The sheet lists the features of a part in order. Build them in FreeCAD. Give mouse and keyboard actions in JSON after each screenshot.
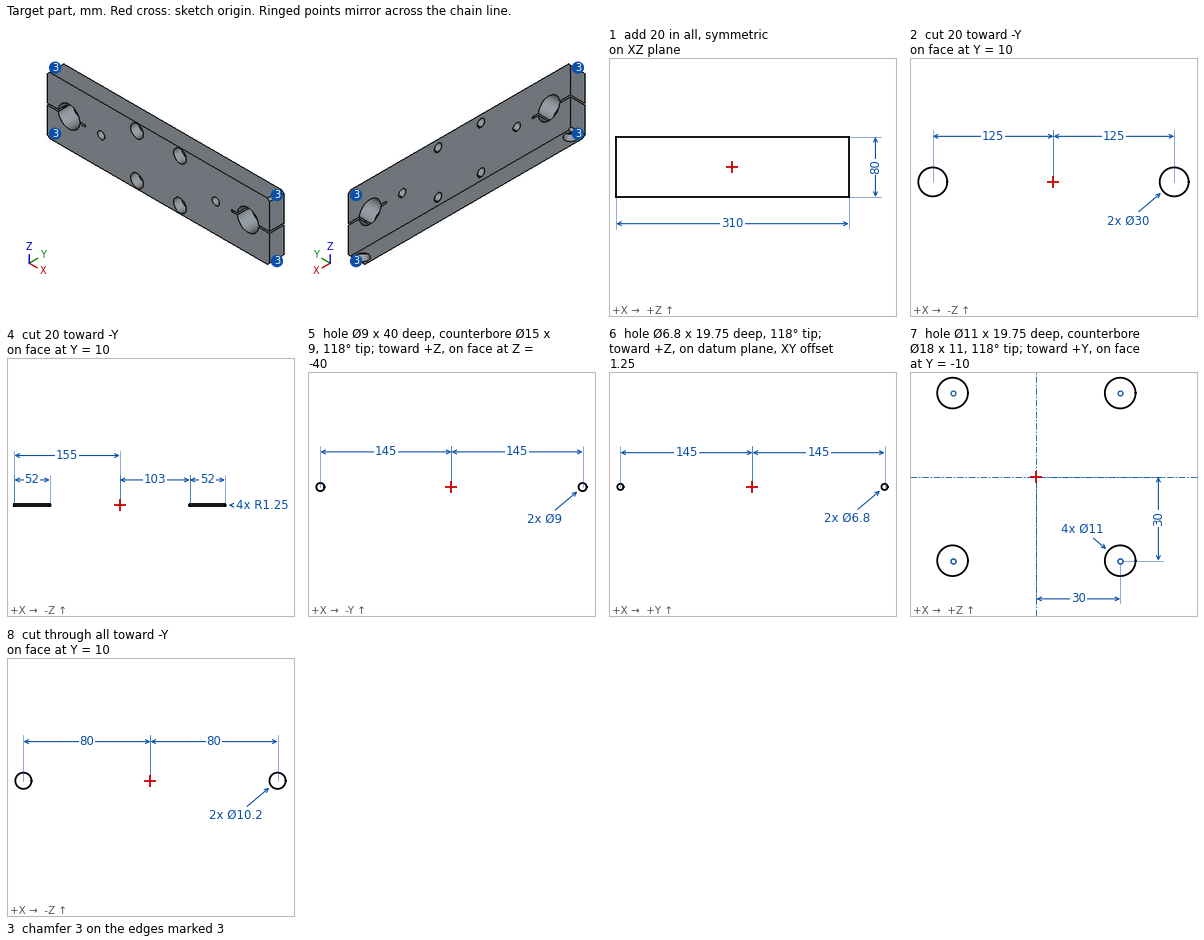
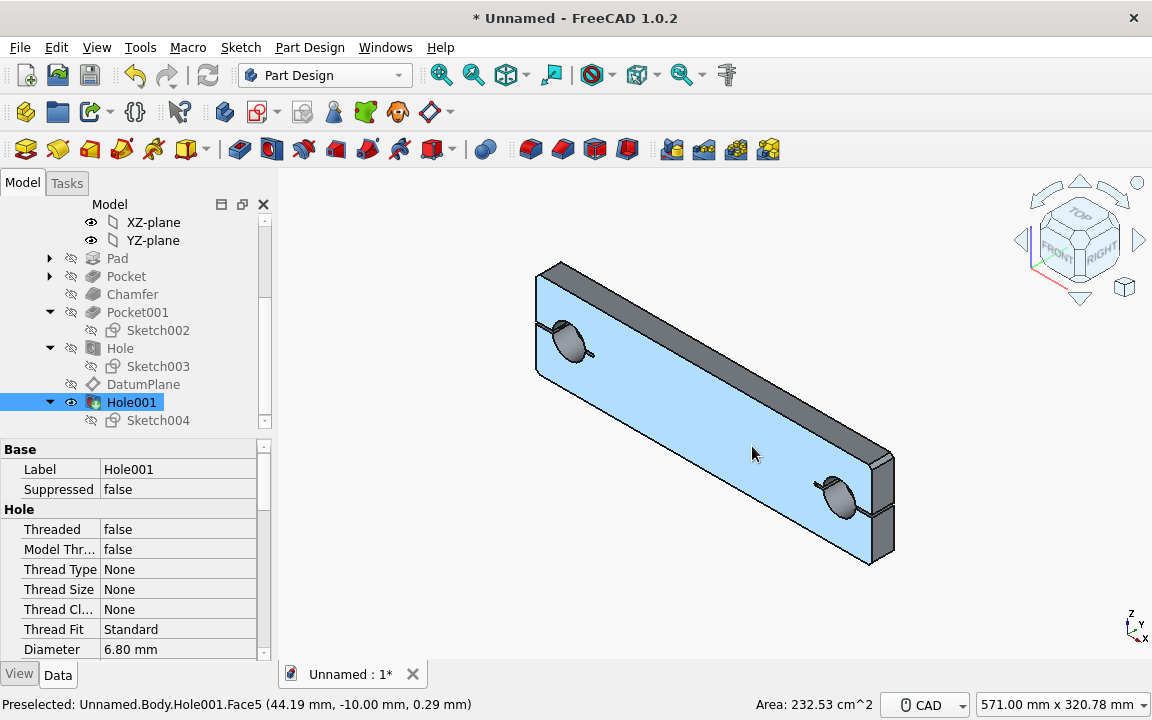
{"action": "left_click", "coordinate": [258, 112]}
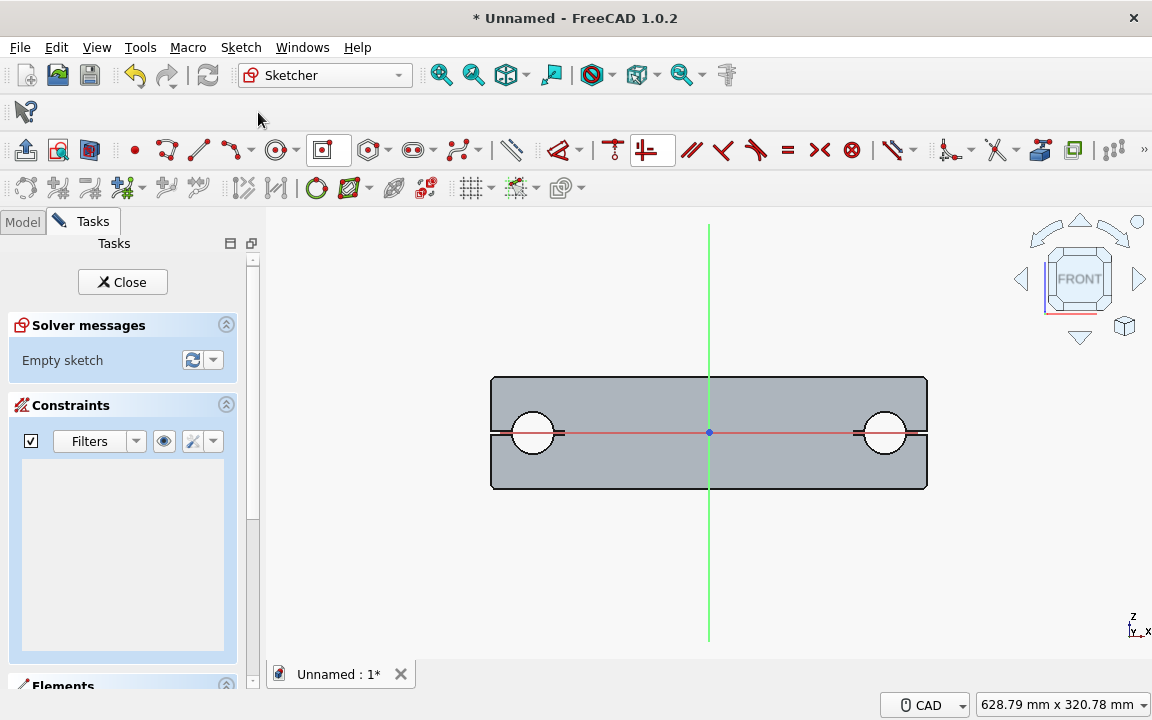
{"action": "scroll", "coordinate": [749, 433], "scroll_direction": "up", "scroll_amount": 5}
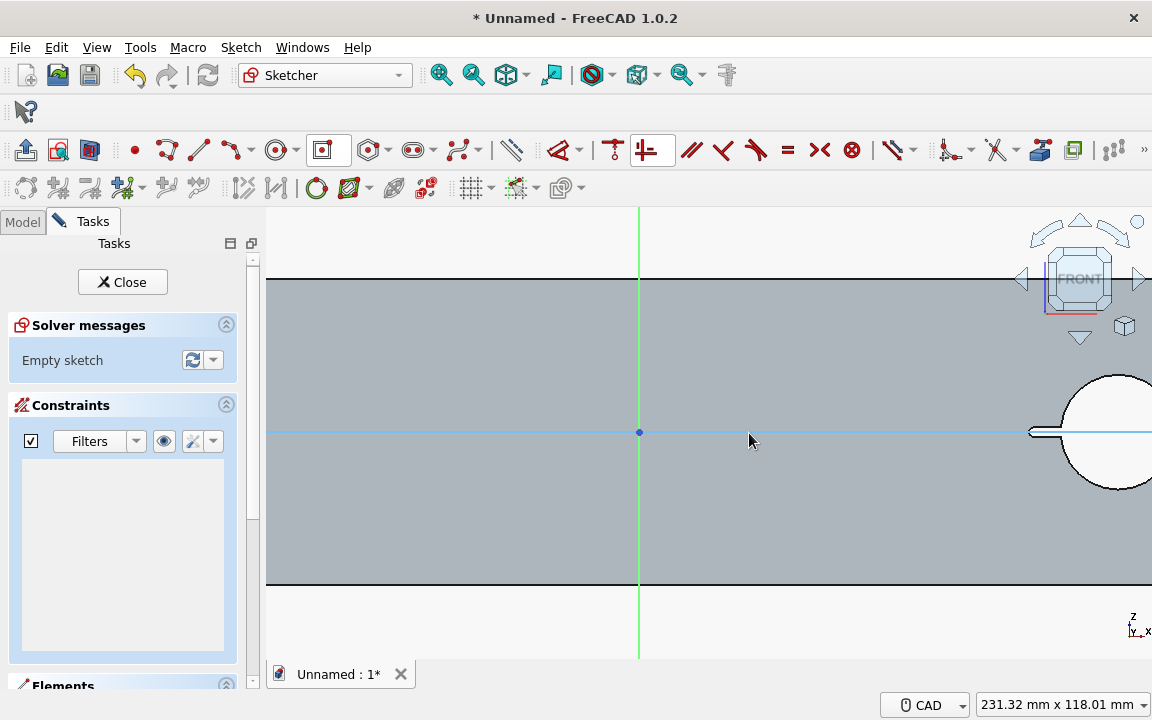
{"action": "left_click", "coordinate": [276, 150]}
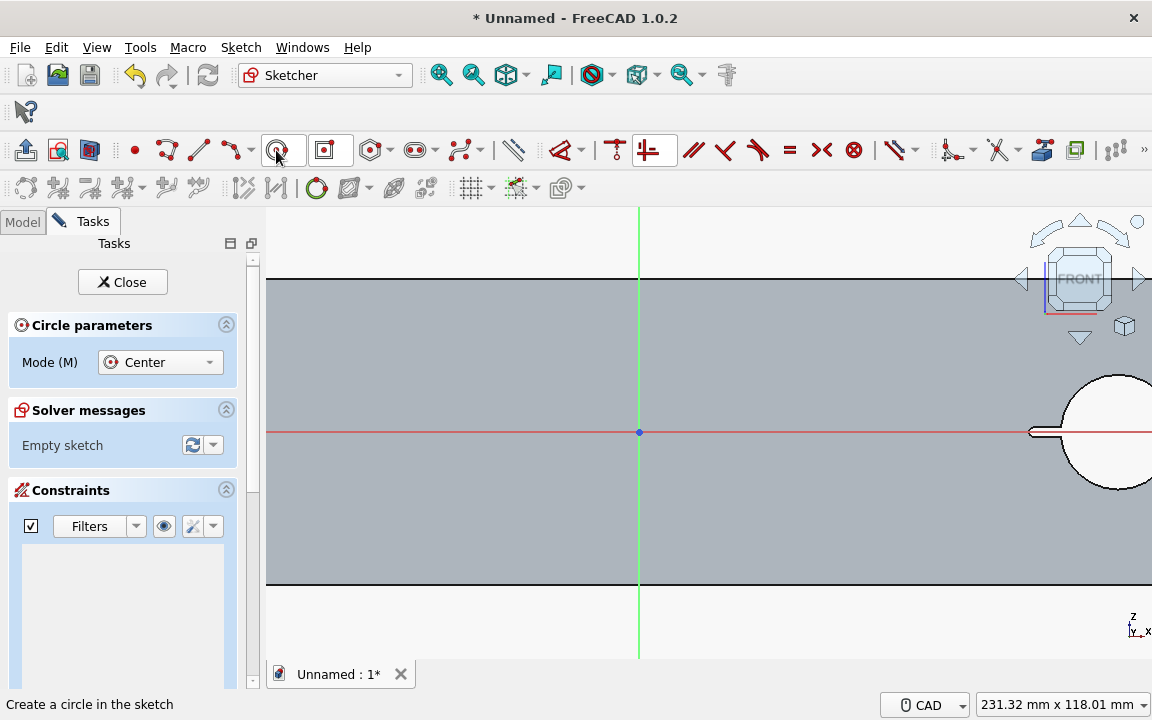
{"action": "left_click", "coordinate": [754, 547]}
{"action": "mouse_move", "coordinate": [769, 532]}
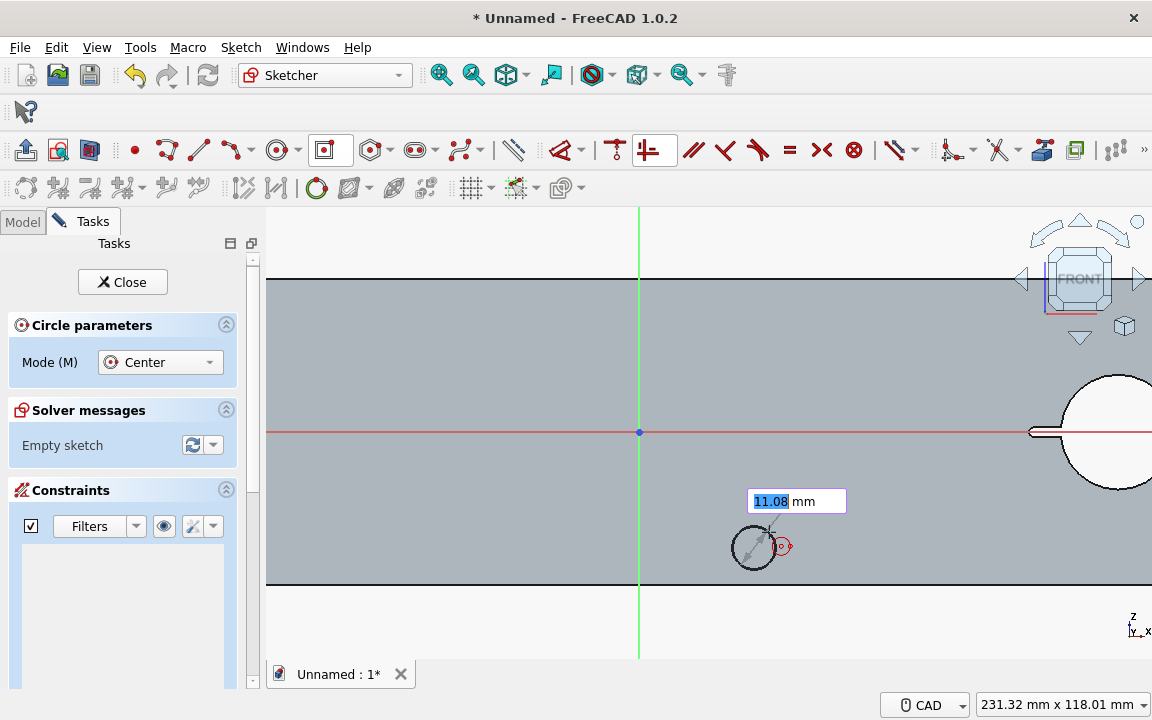
{"action": "type", "text": "11"}
{"action": "key", "text": "Return"}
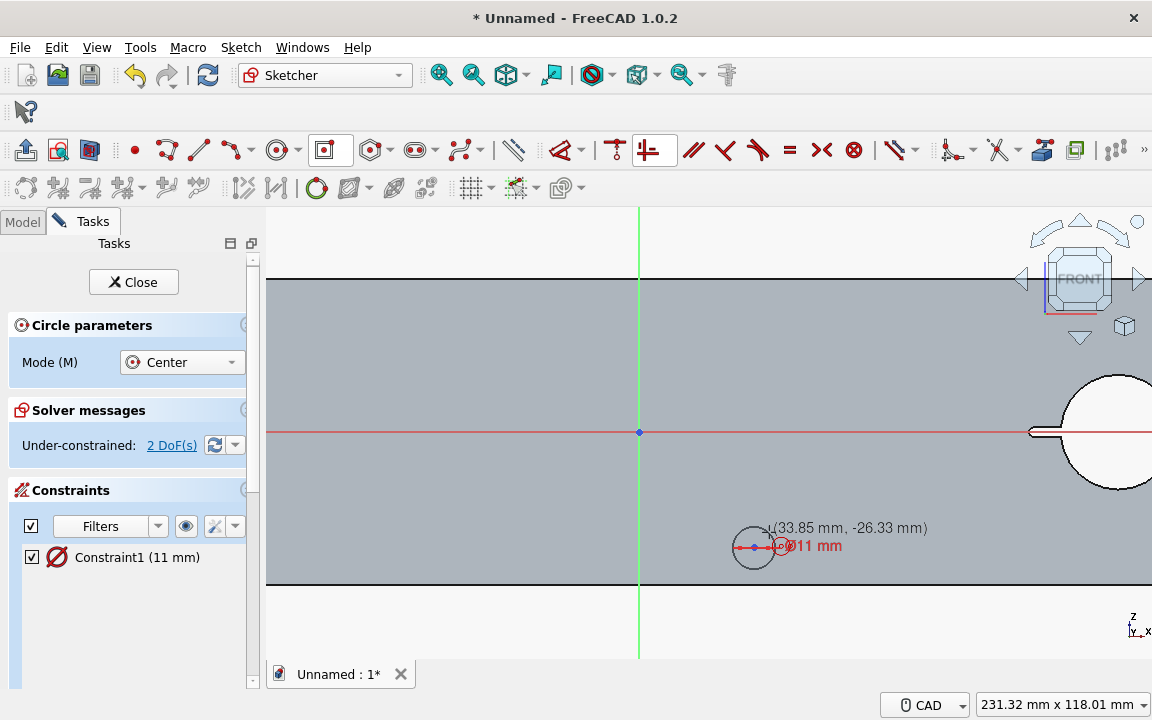
{"action": "left_click", "coordinate": [524, 547]}
{"action": "mouse_move", "coordinate": [539, 532]}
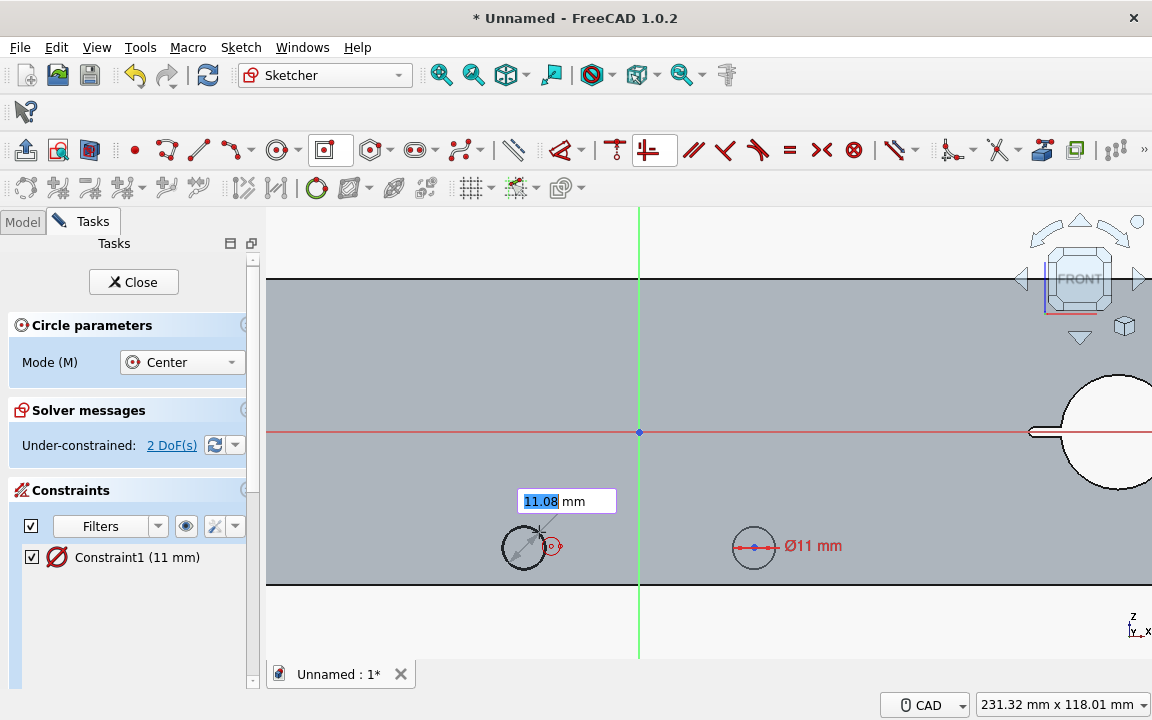
{"action": "type", "text": "11"}
{"action": "key", "text": "Return"}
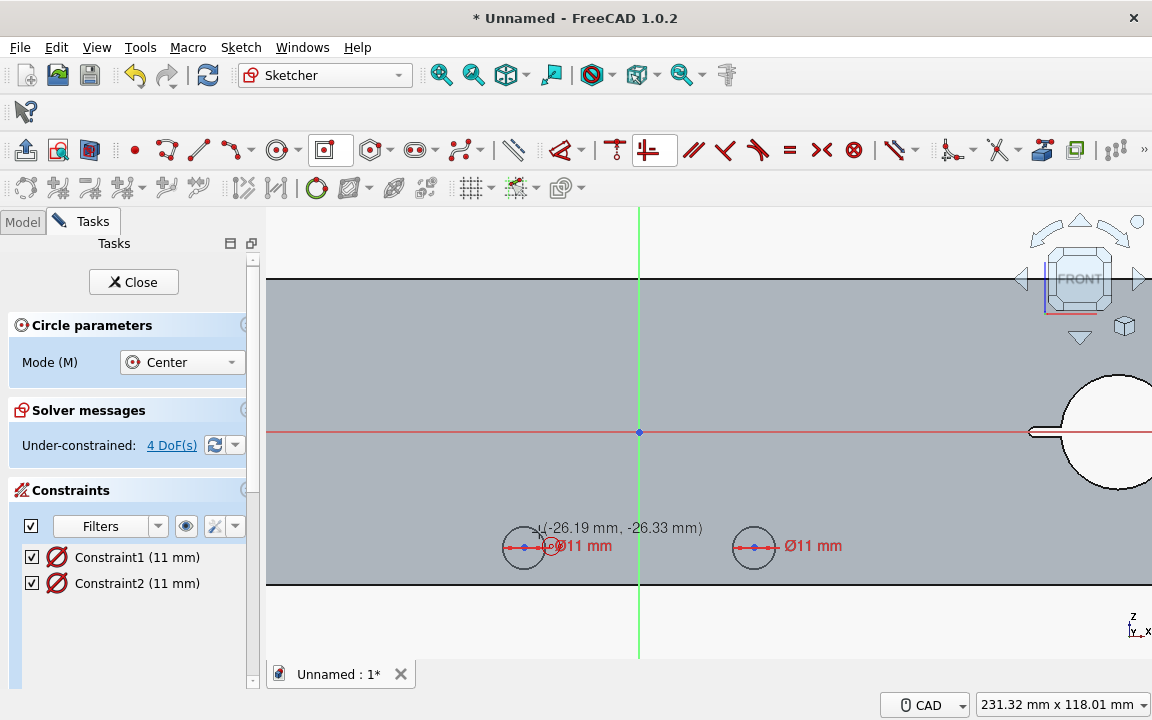
{"action": "left_click", "coordinate": [524, 317]}
{"action": "mouse_move", "coordinate": [539, 302]}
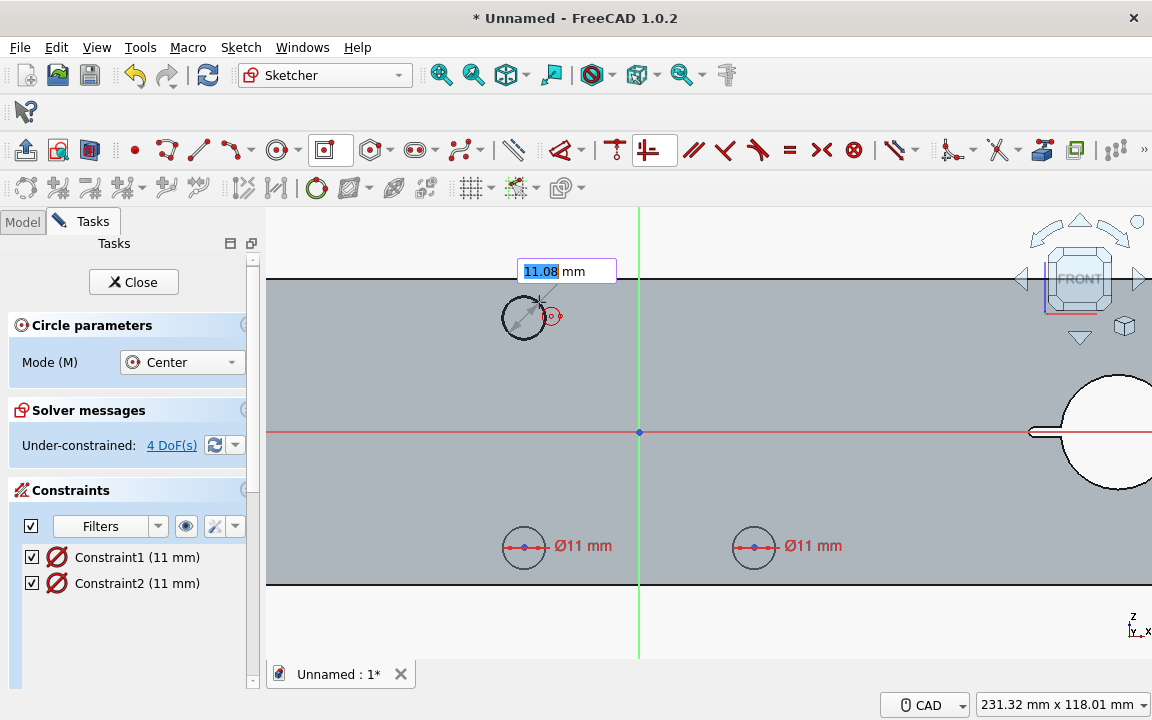
{"action": "type", "text": "11"}
{"action": "key", "text": "Return"}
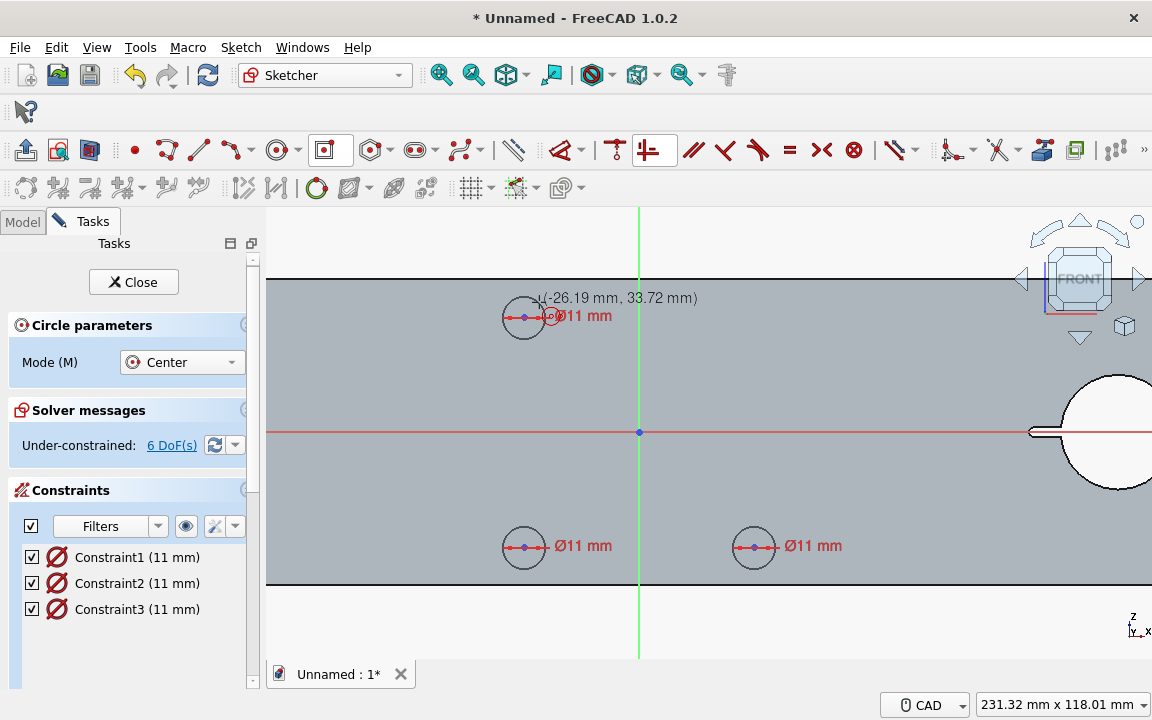
{"action": "left_click", "coordinate": [754, 317]}
{"action": "mouse_move", "coordinate": [769, 302]}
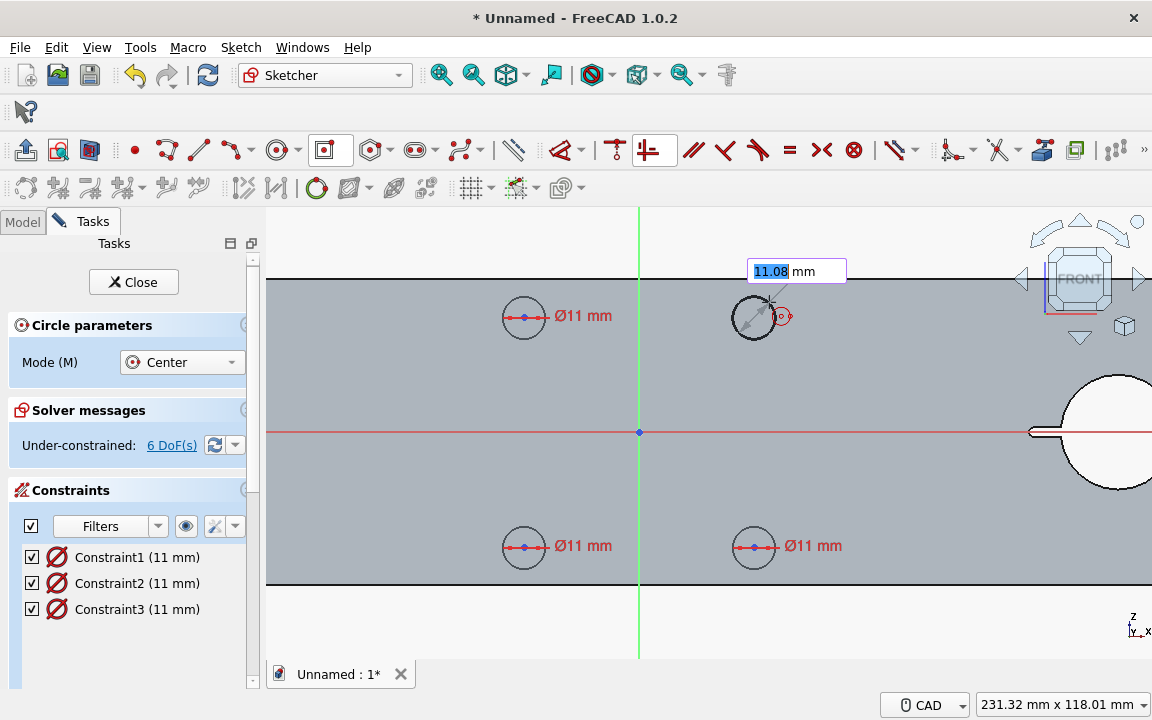
{"action": "type", "text": "11"}
{"action": "key", "text": "Return"}
{"action": "key", "text": "Escape"}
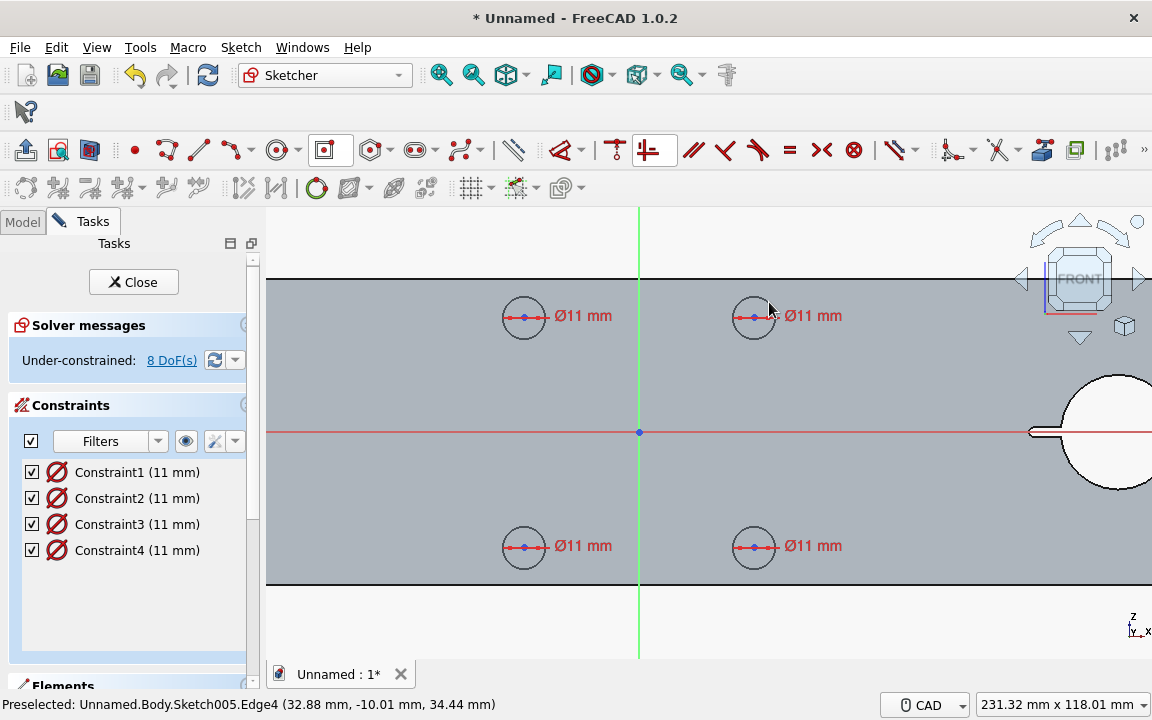
{"action": "left_click", "coordinate": [754, 548]}